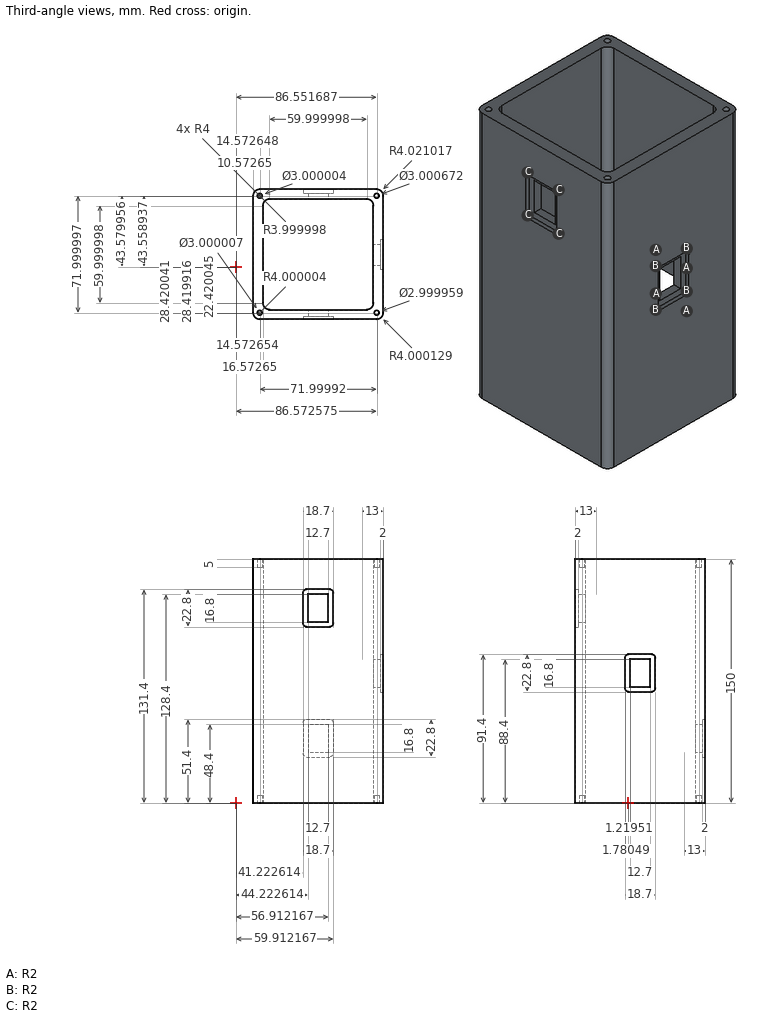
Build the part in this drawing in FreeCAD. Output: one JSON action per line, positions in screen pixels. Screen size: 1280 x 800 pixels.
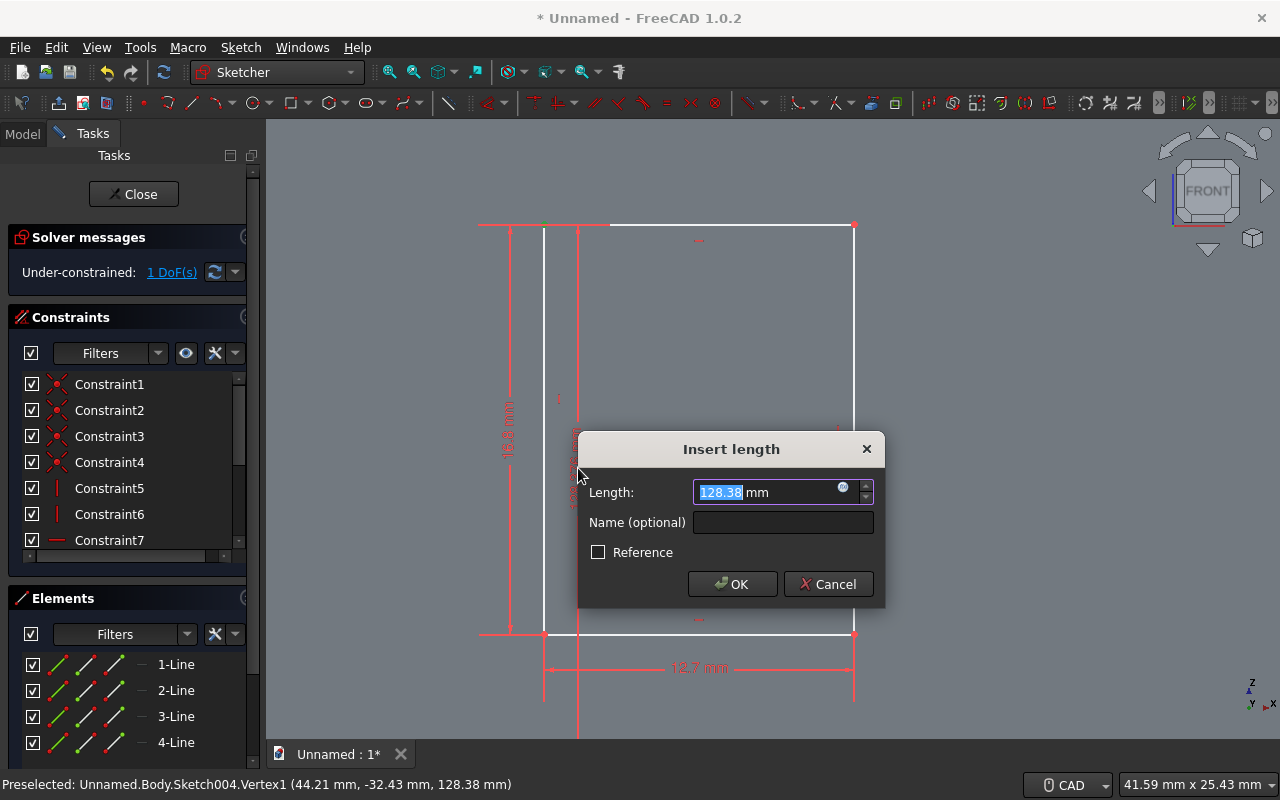
{"action": "type", "text": "128.4"}
{"action": "key", "text": "Return"}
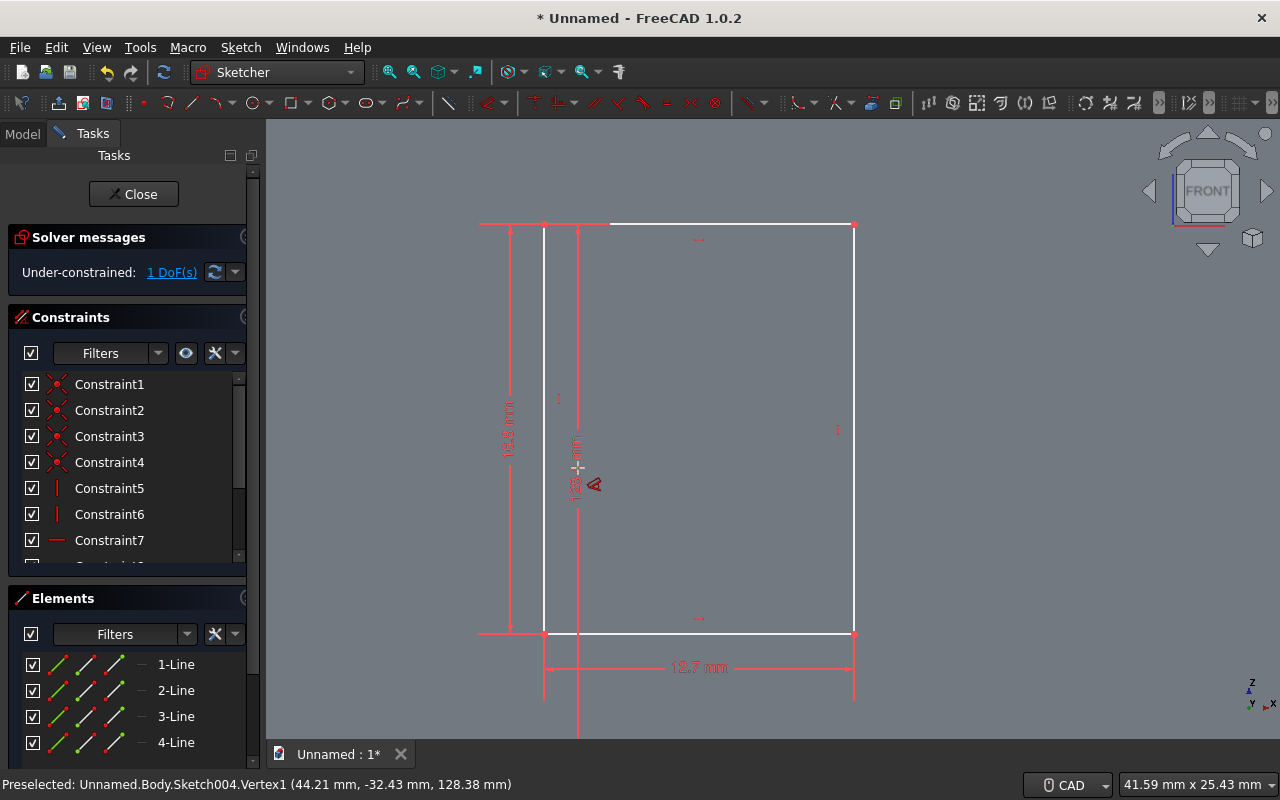
{"action": "left_click", "coordinate": [544, 224]}
{"action": "left_click", "coordinate": [419, 190]}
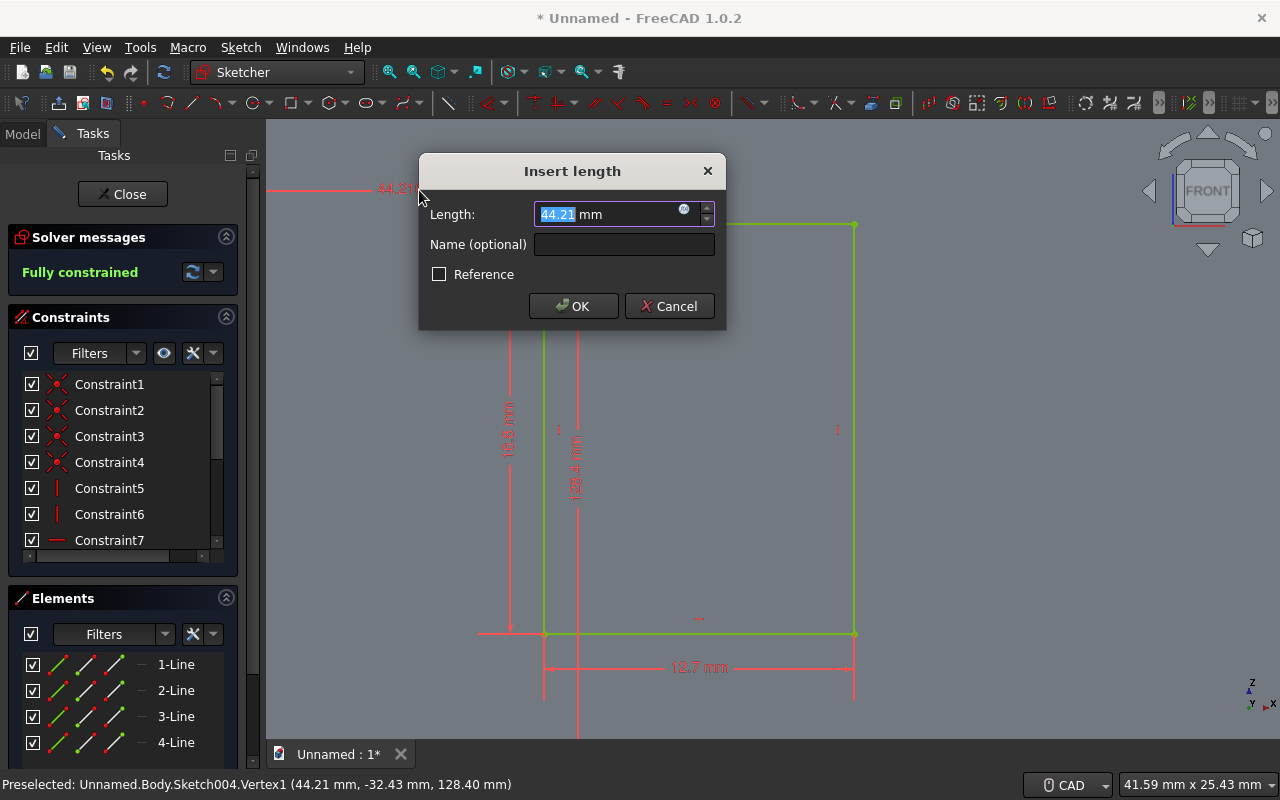
{"action": "type", "text": "44.222614"}
{"action": "key", "text": "Return"}
{"action": "key", "text": "Escape"}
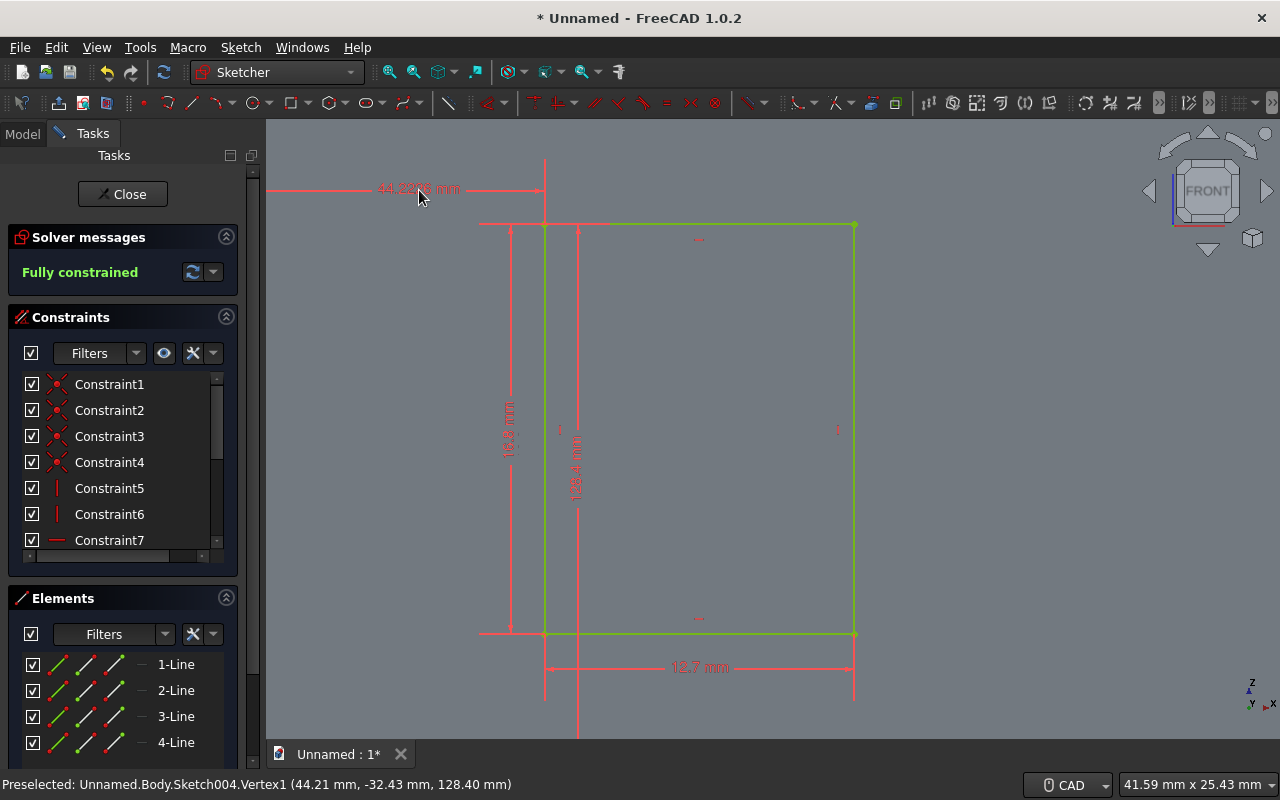
{"action": "left_click", "coordinate": [123, 194]}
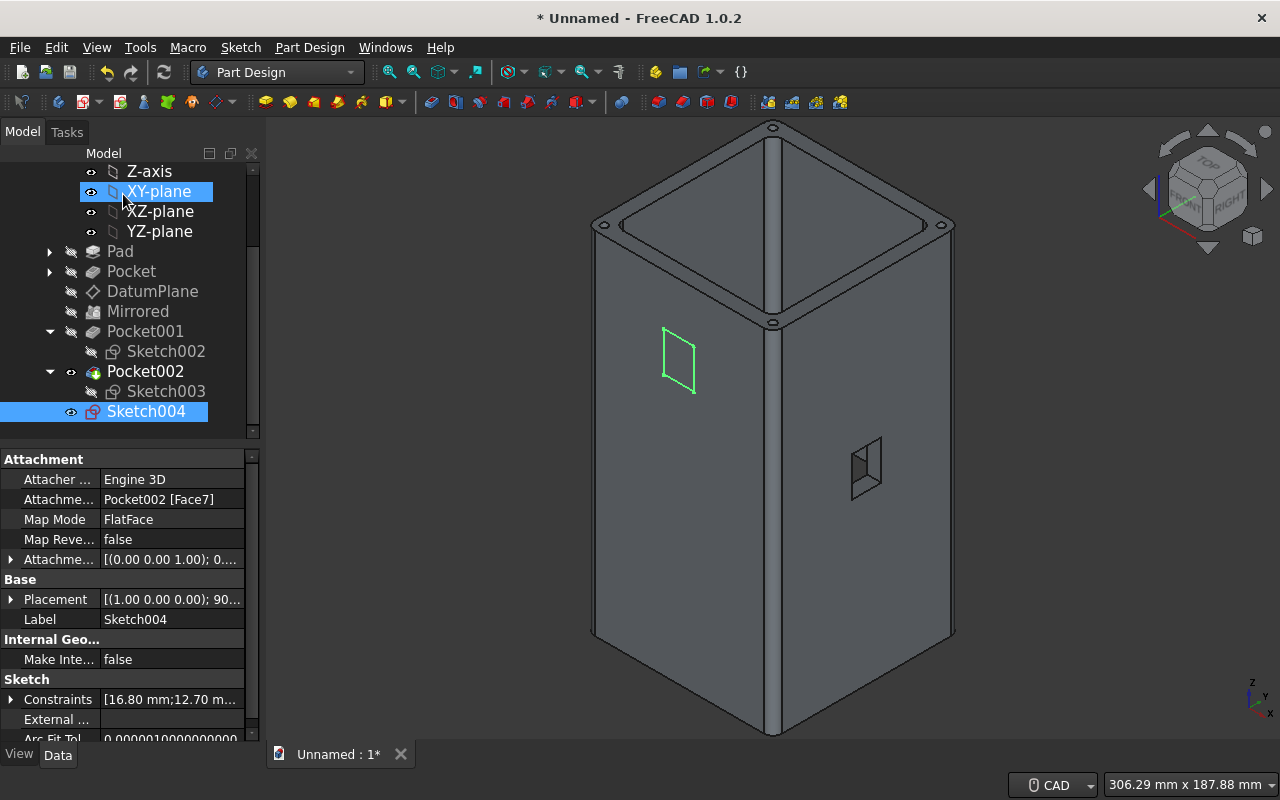
{"action": "left_click", "coordinate": [432, 102]}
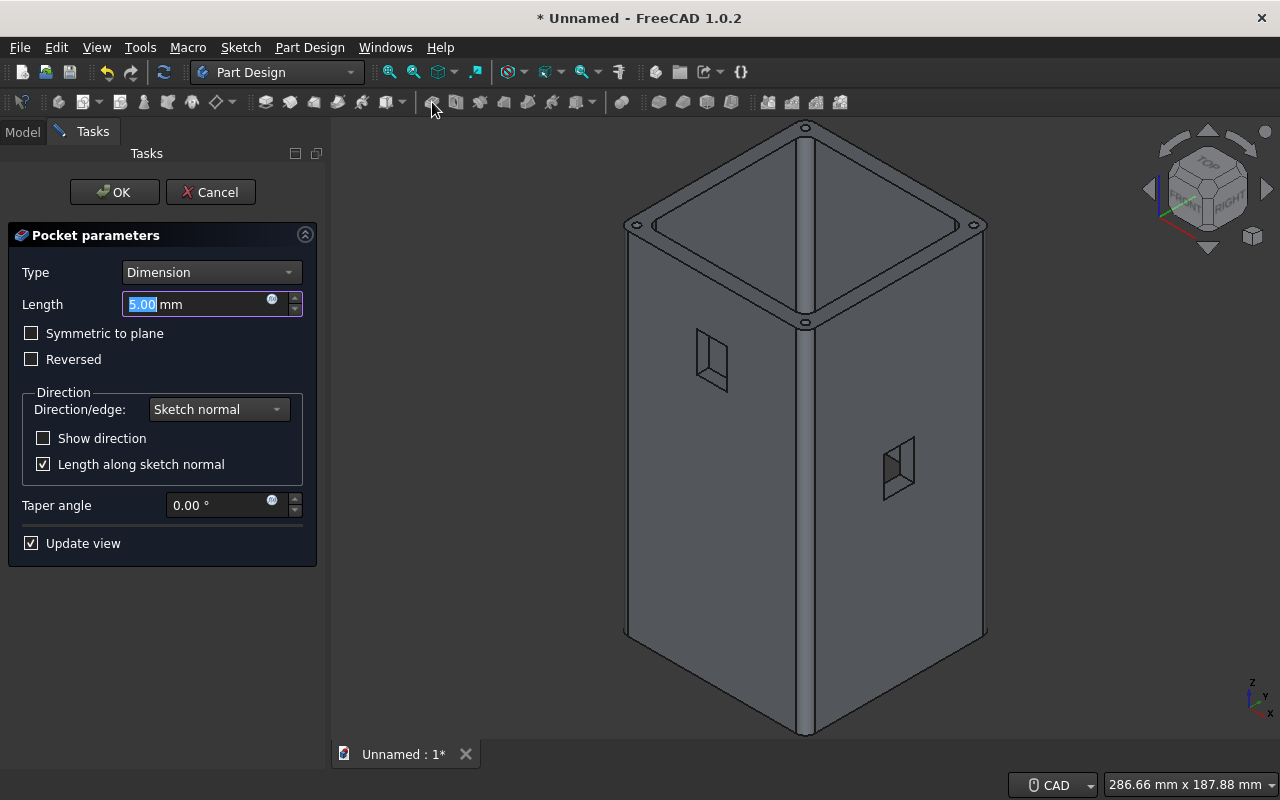
{"action": "type", "text": "13"}
{"action": "key", "text": "Tab"}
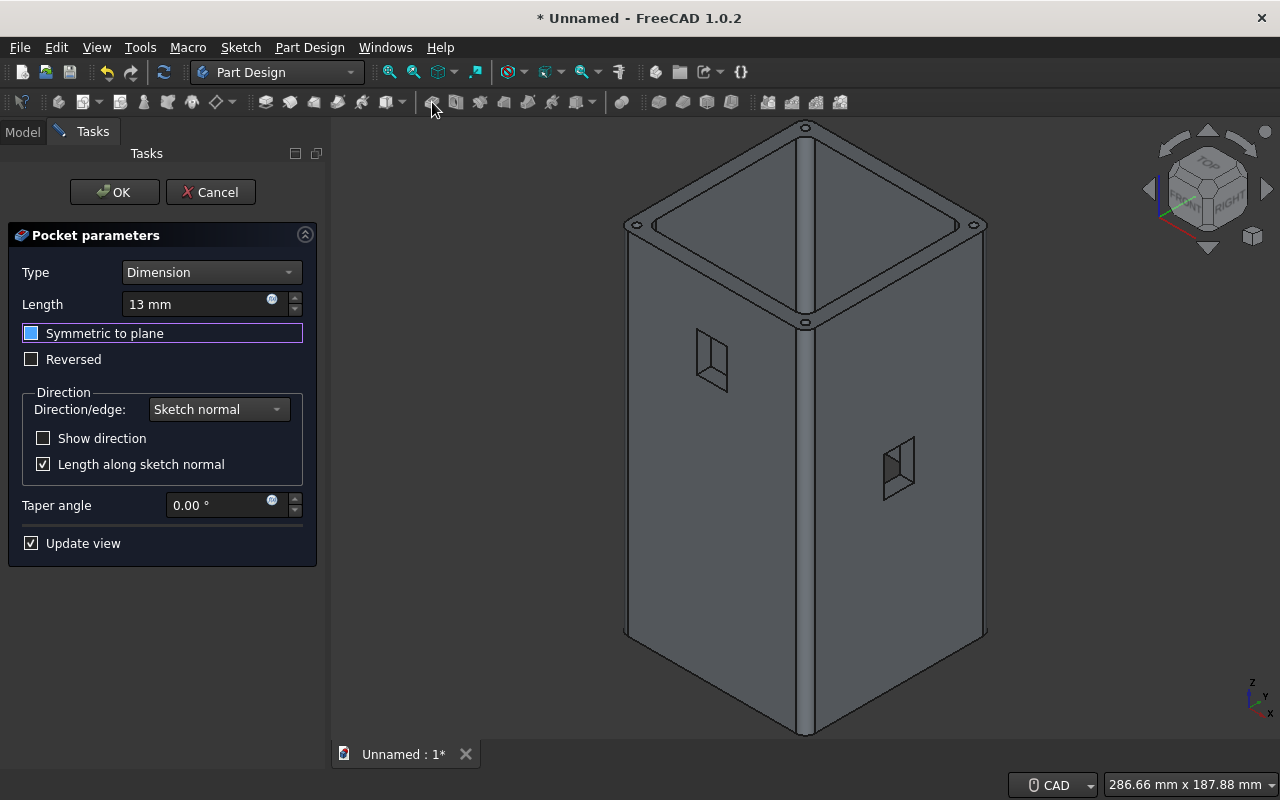
{"action": "left_click", "coordinate": [115, 192]}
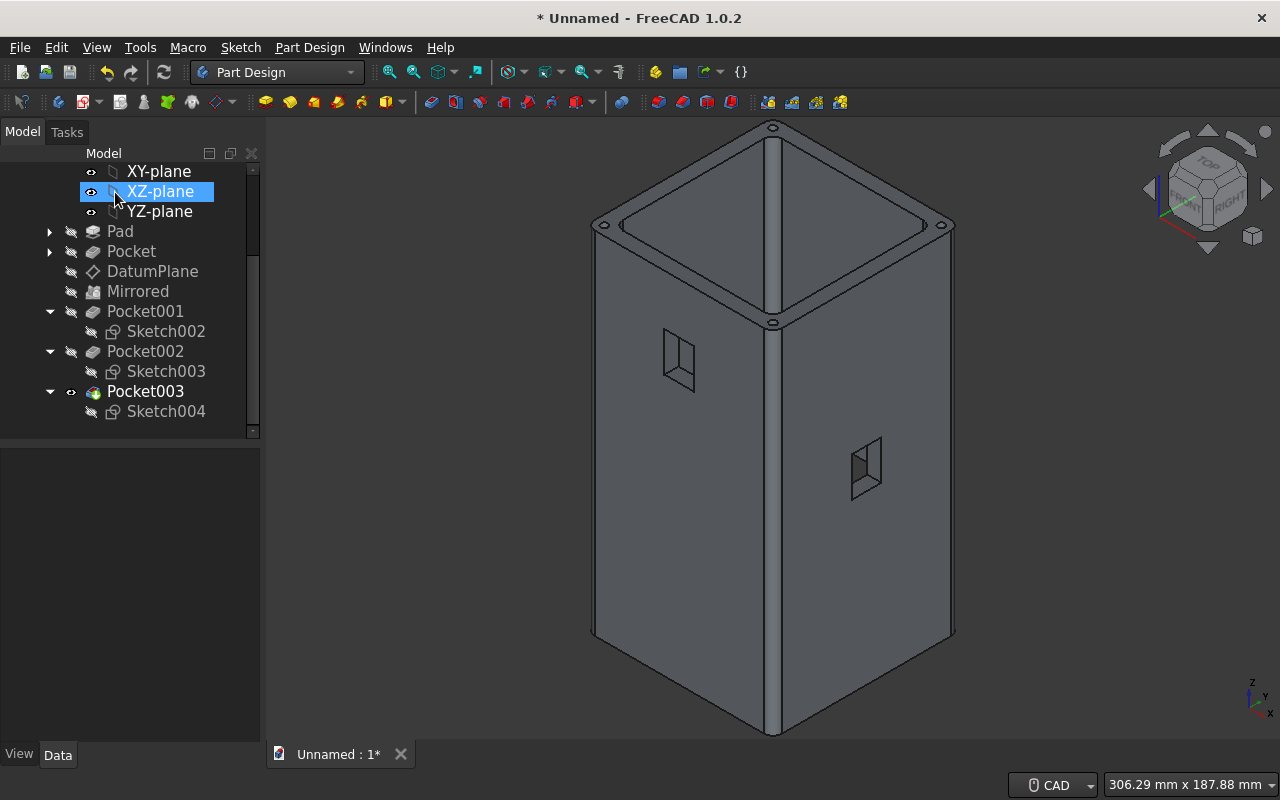
{"action": "left_click", "coordinate": [390, 72]}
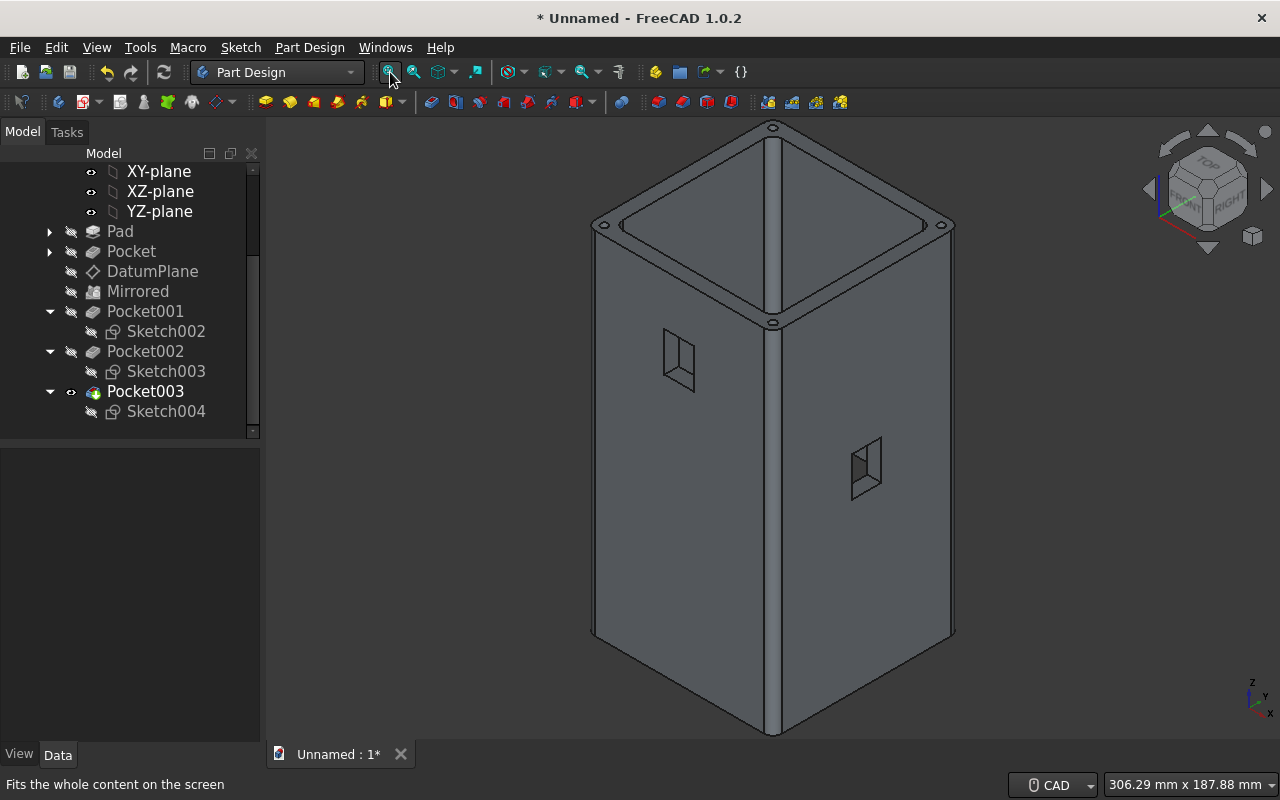
{"action": "key", "text": "4"}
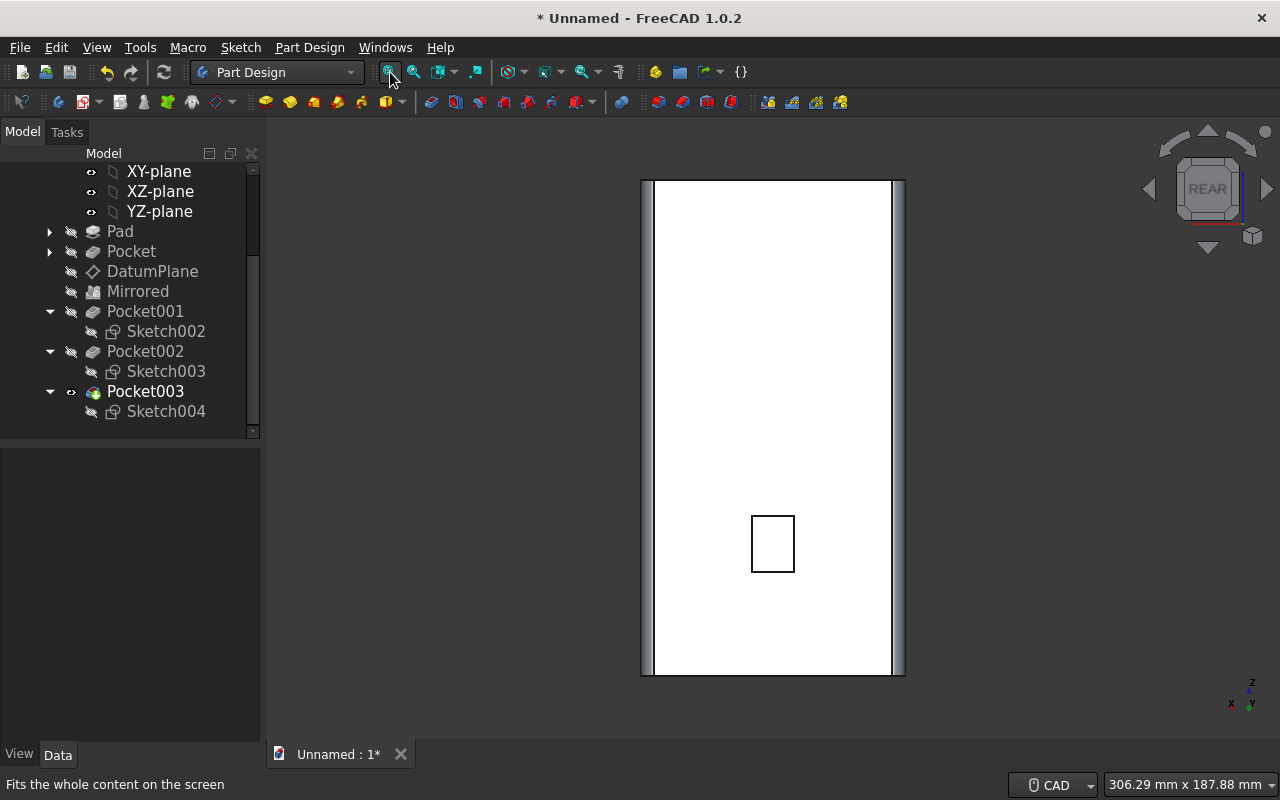
{"action": "left_click", "coordinate": [773, 356]}